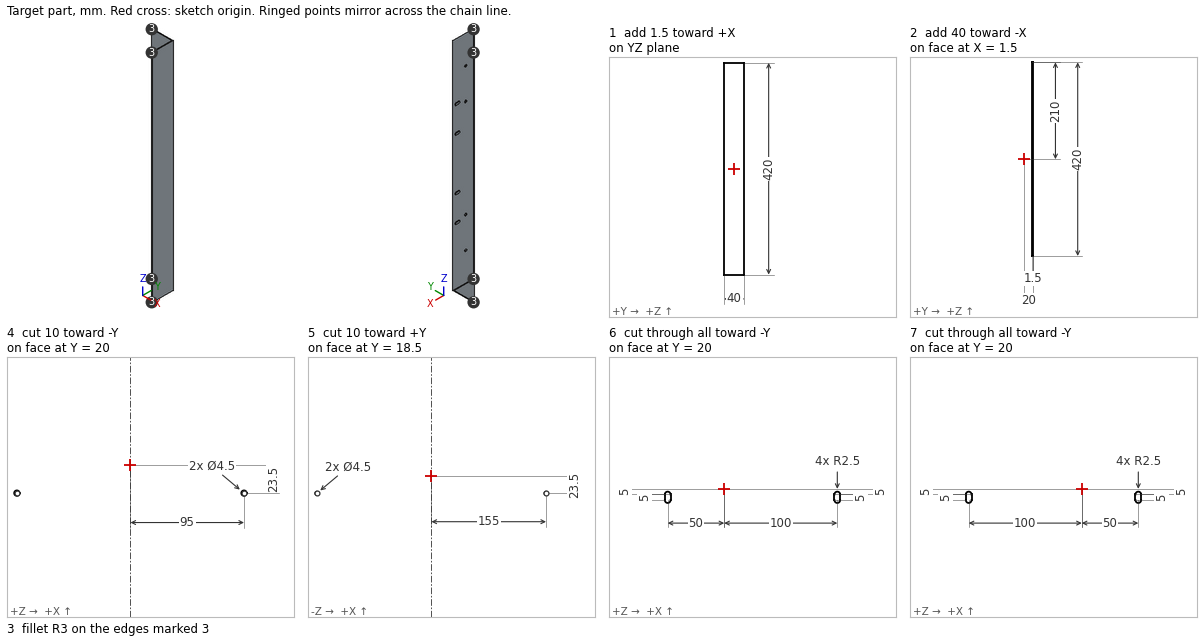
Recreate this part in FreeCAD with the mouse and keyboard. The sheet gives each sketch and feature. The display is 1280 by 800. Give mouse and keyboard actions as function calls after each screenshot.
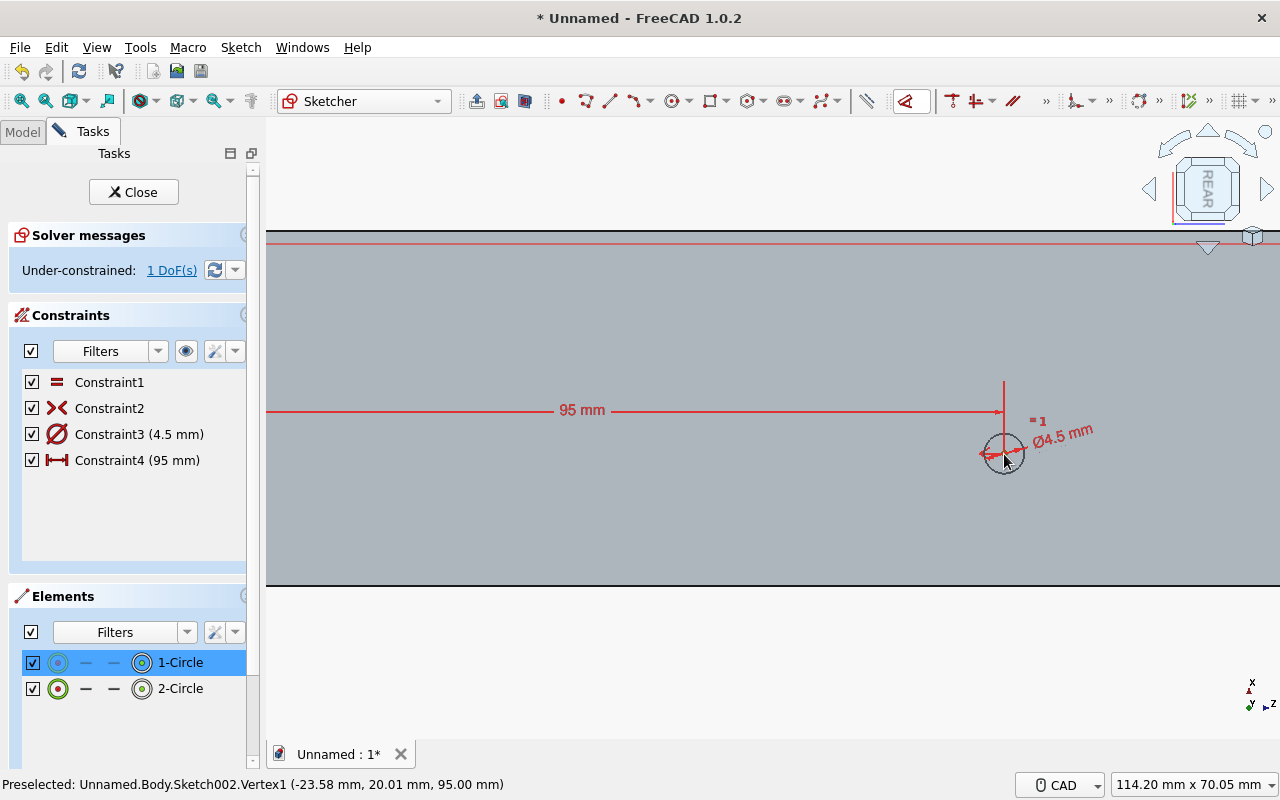
key(i)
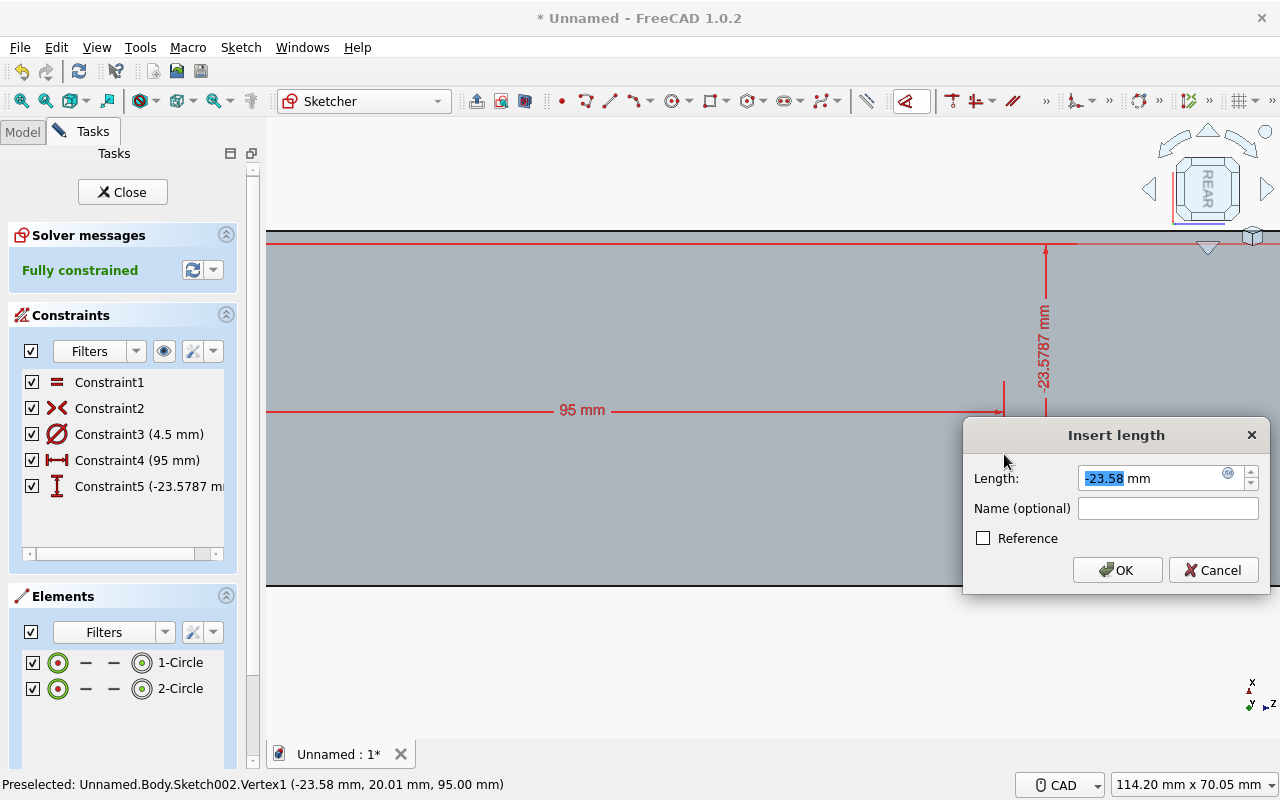
text(-23.5)
key(Return)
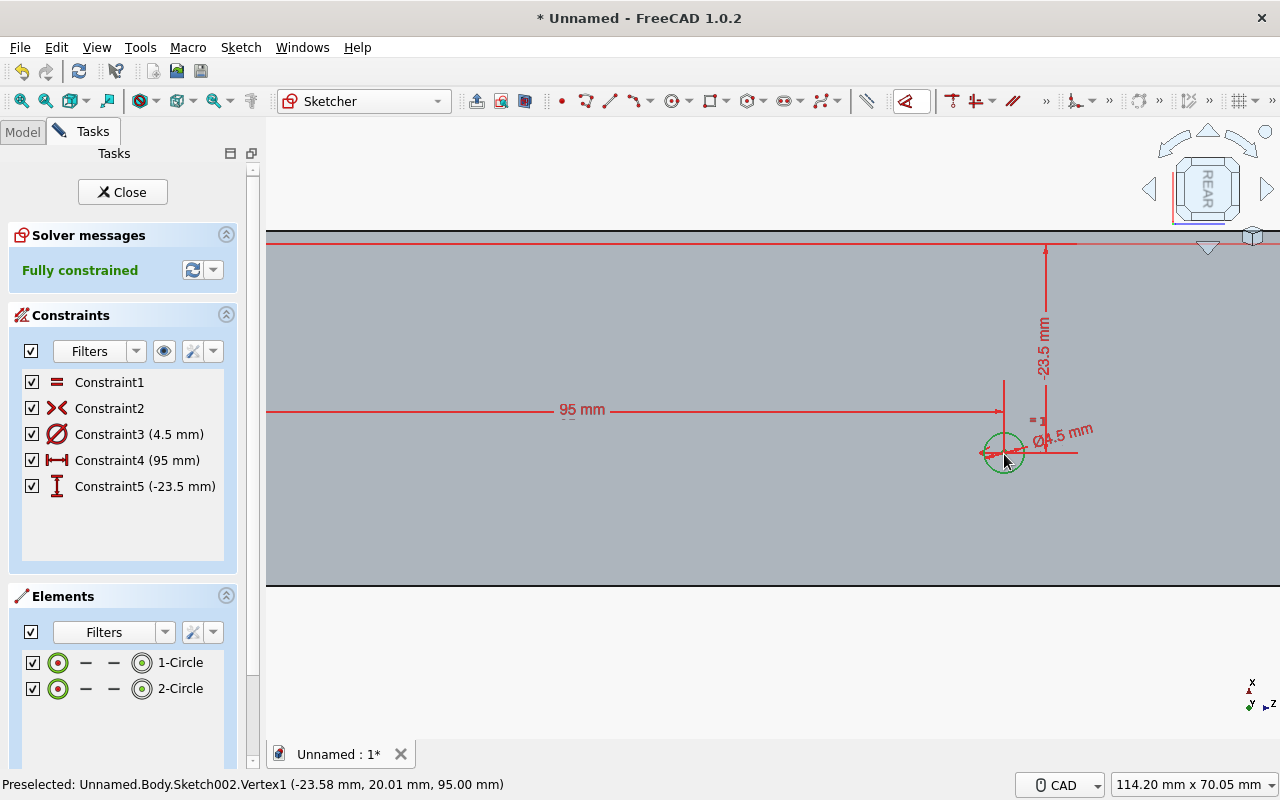
click(123, 192)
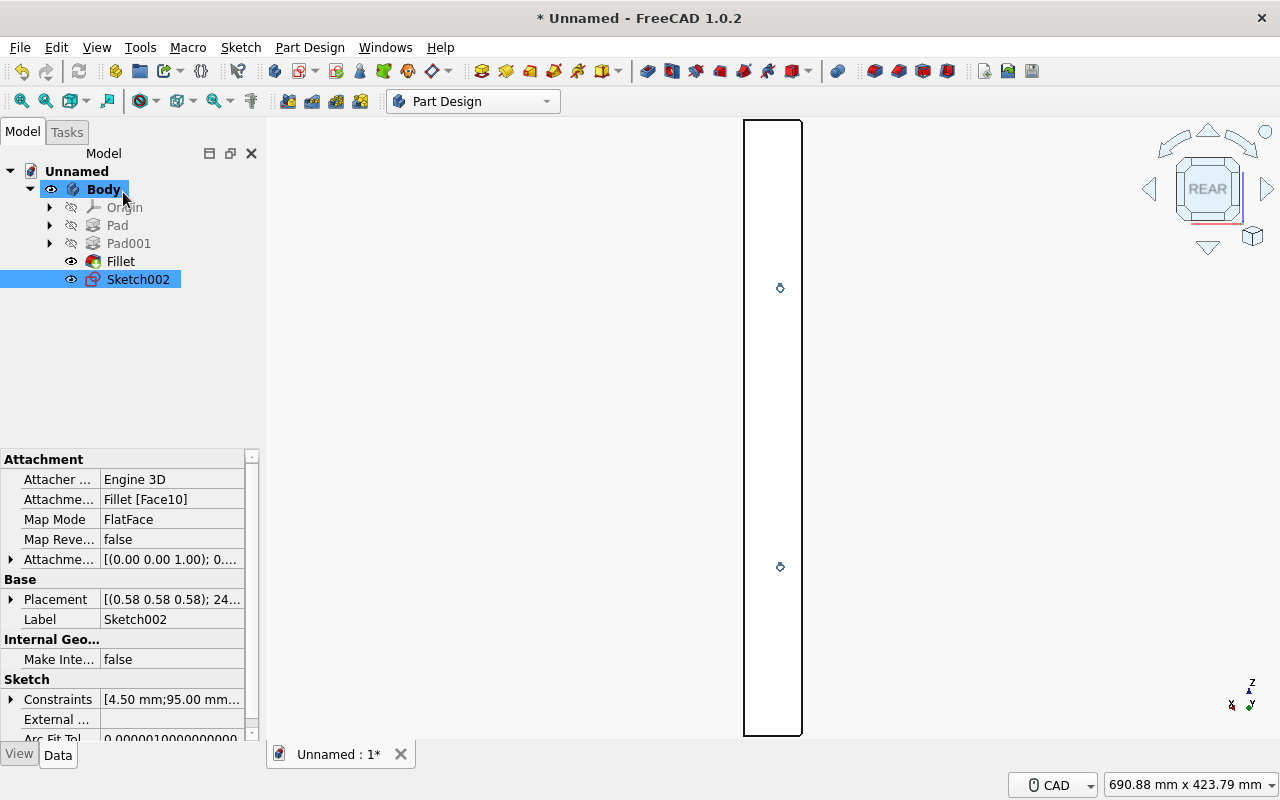
click(648, 72)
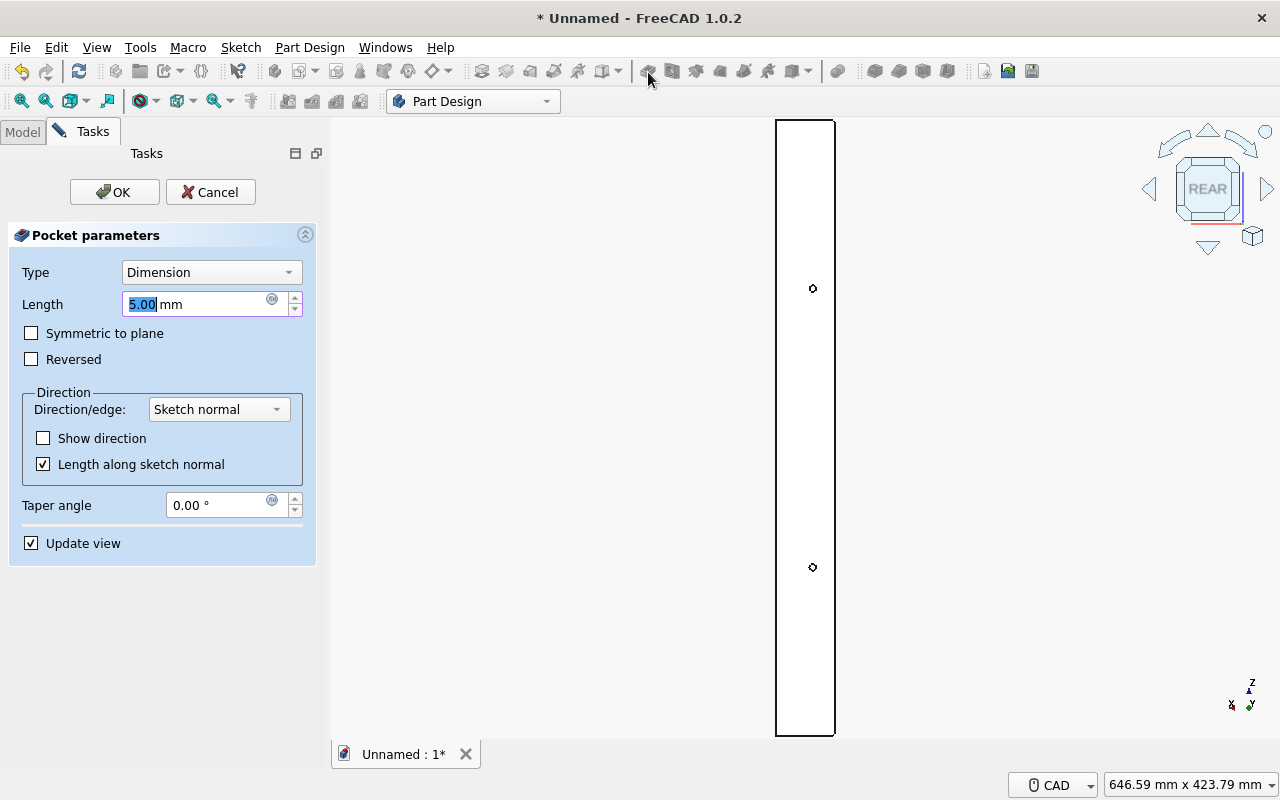
text(10)
key(Tab)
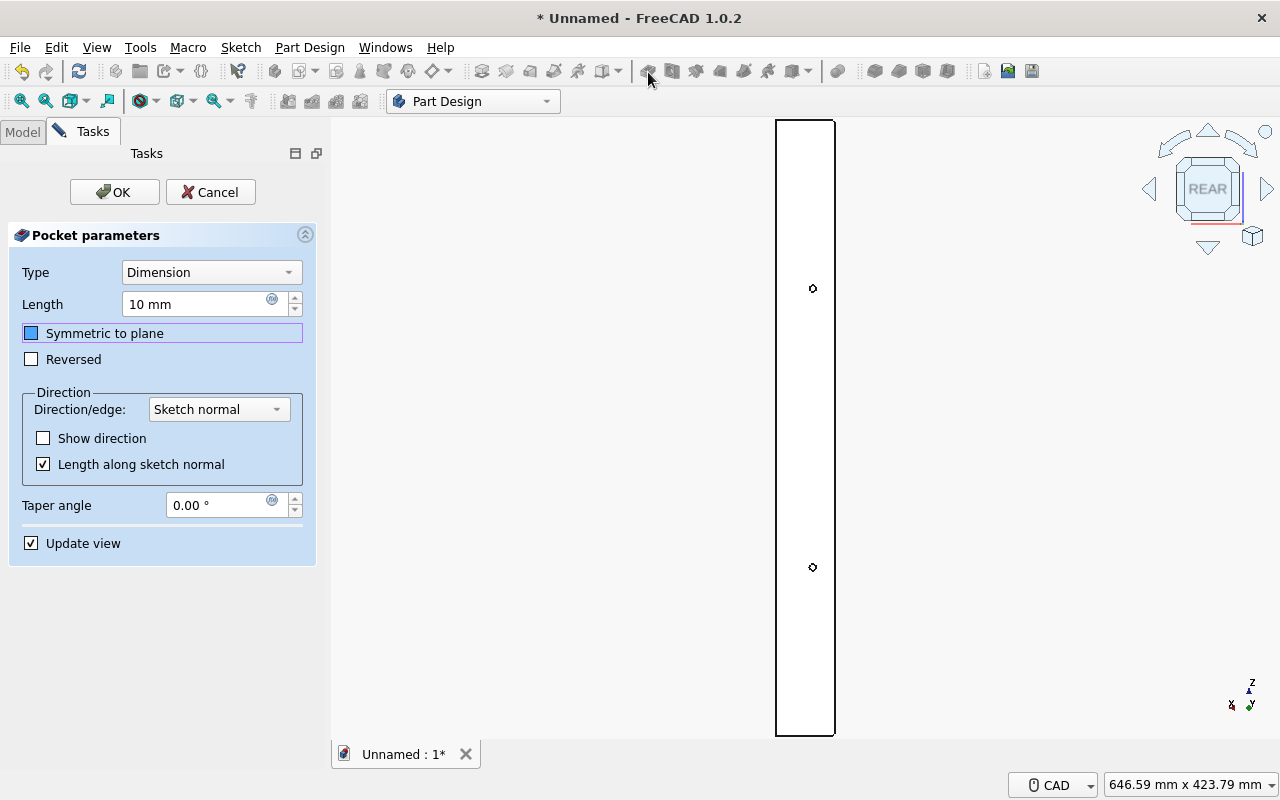
click(115, 192)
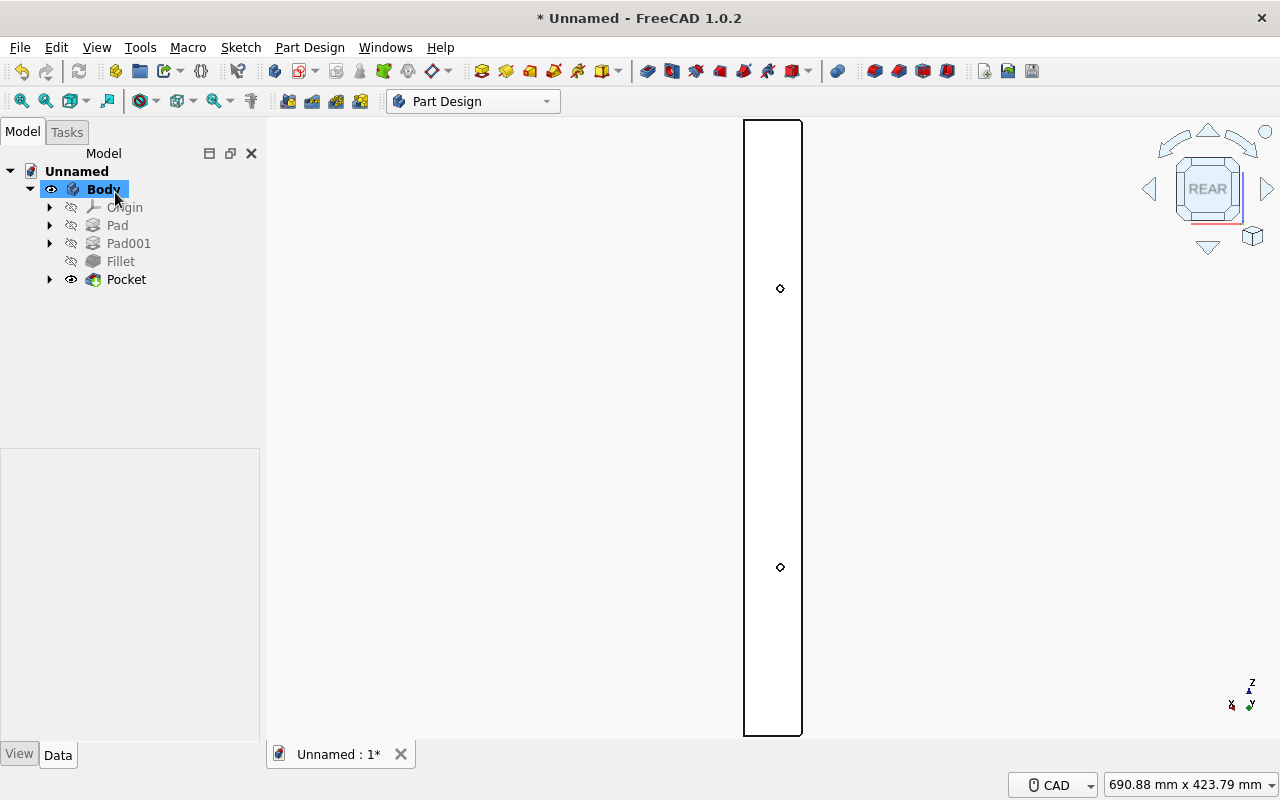
key(0)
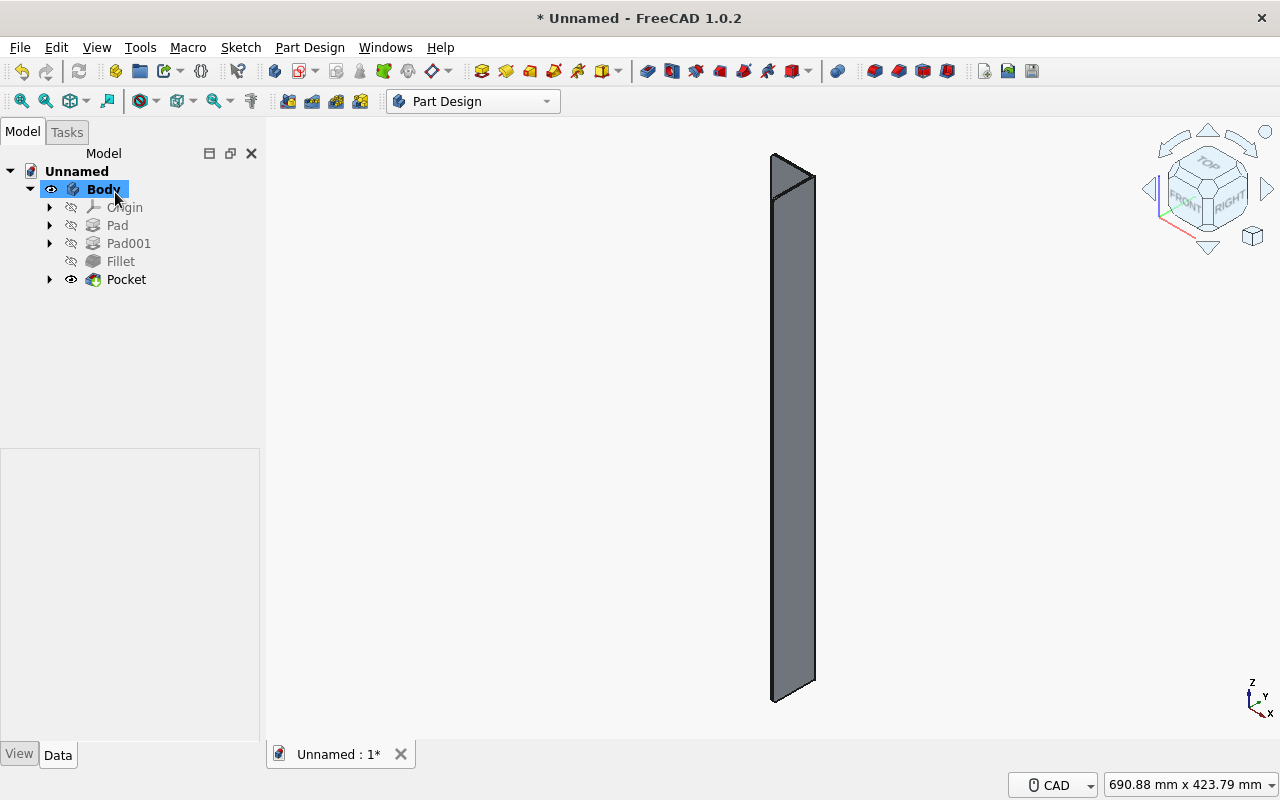
key(1)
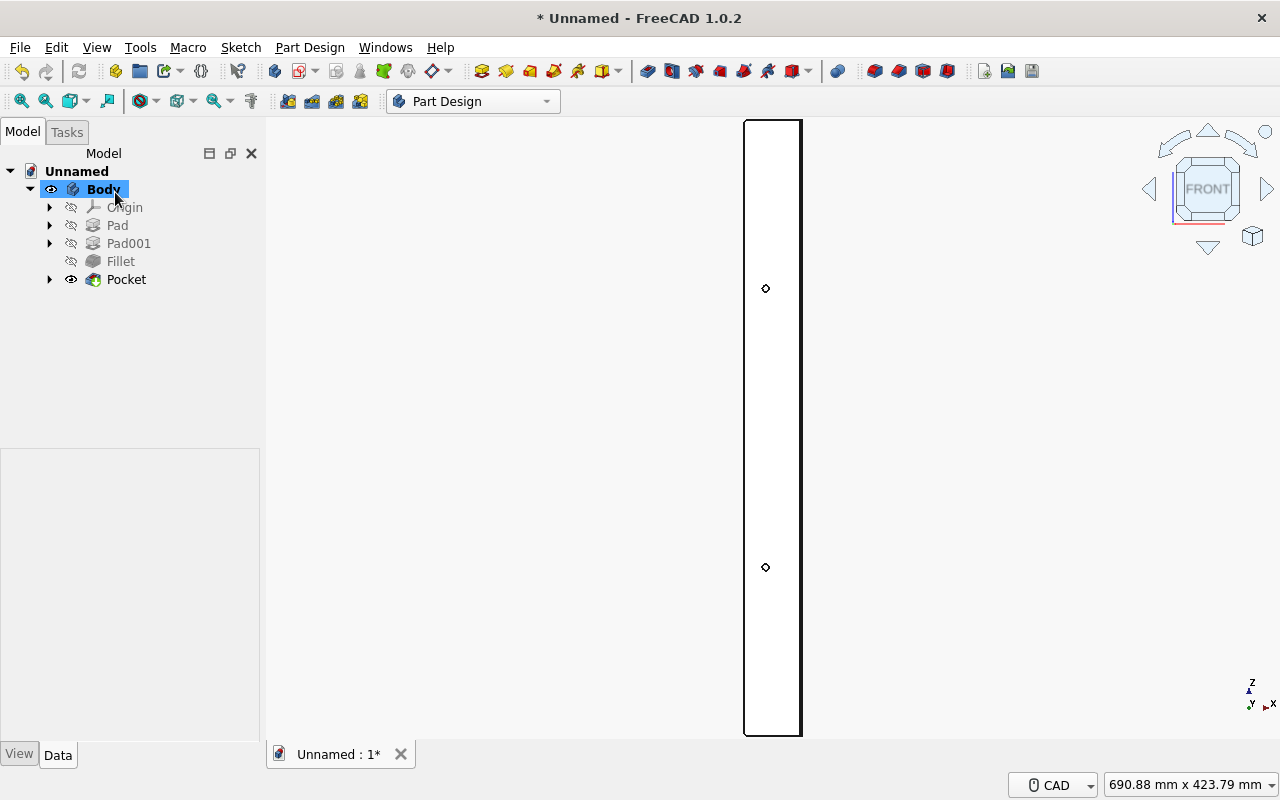
click(772, 251)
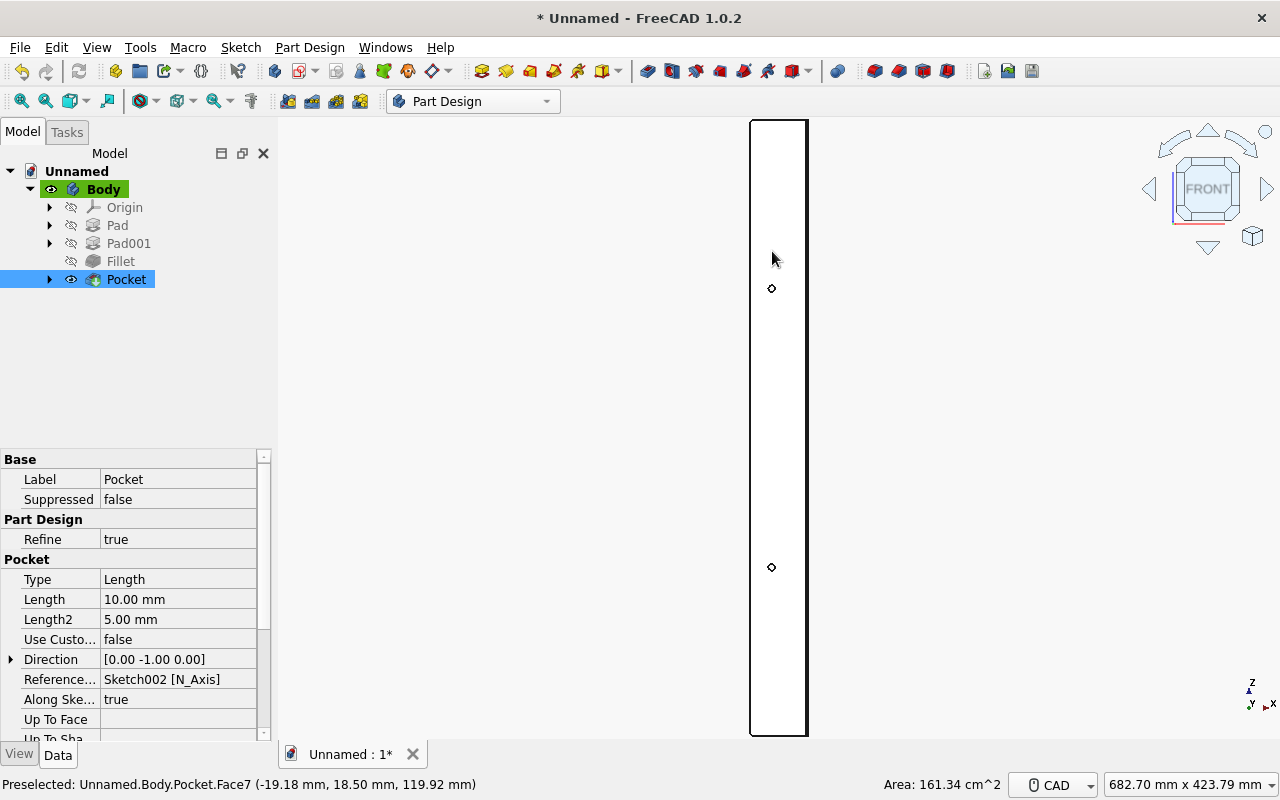
click(300, 72)